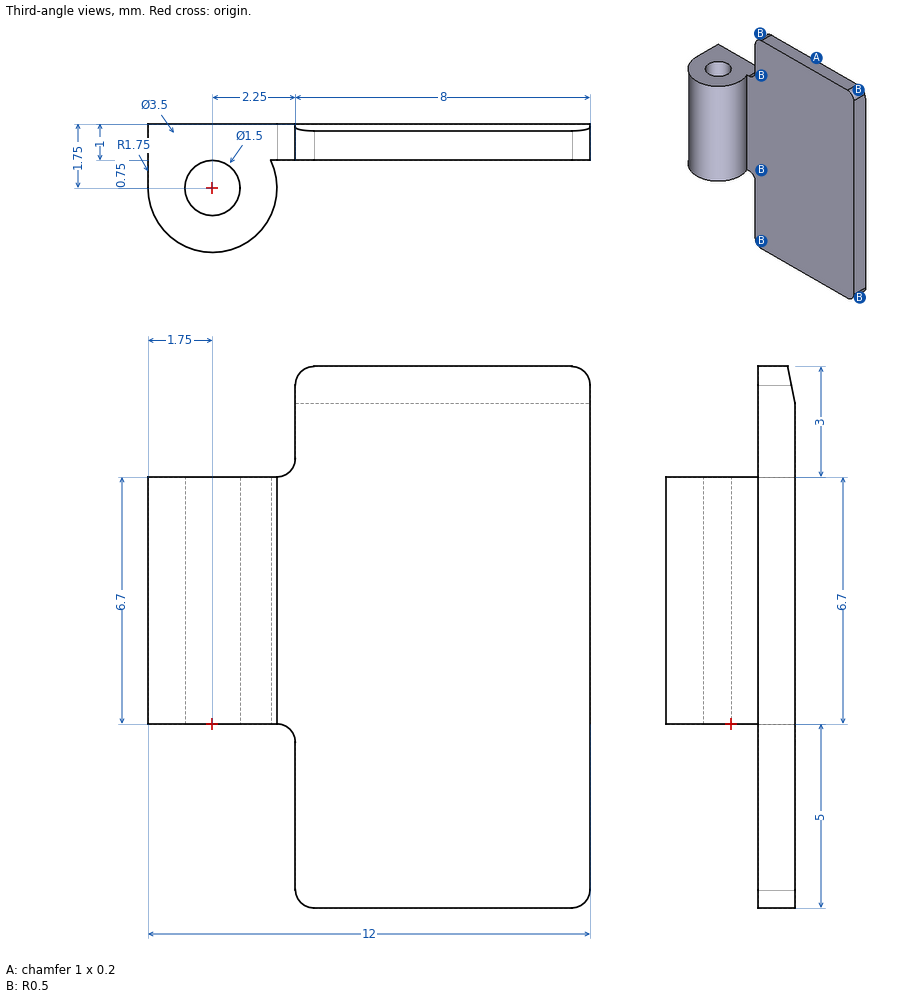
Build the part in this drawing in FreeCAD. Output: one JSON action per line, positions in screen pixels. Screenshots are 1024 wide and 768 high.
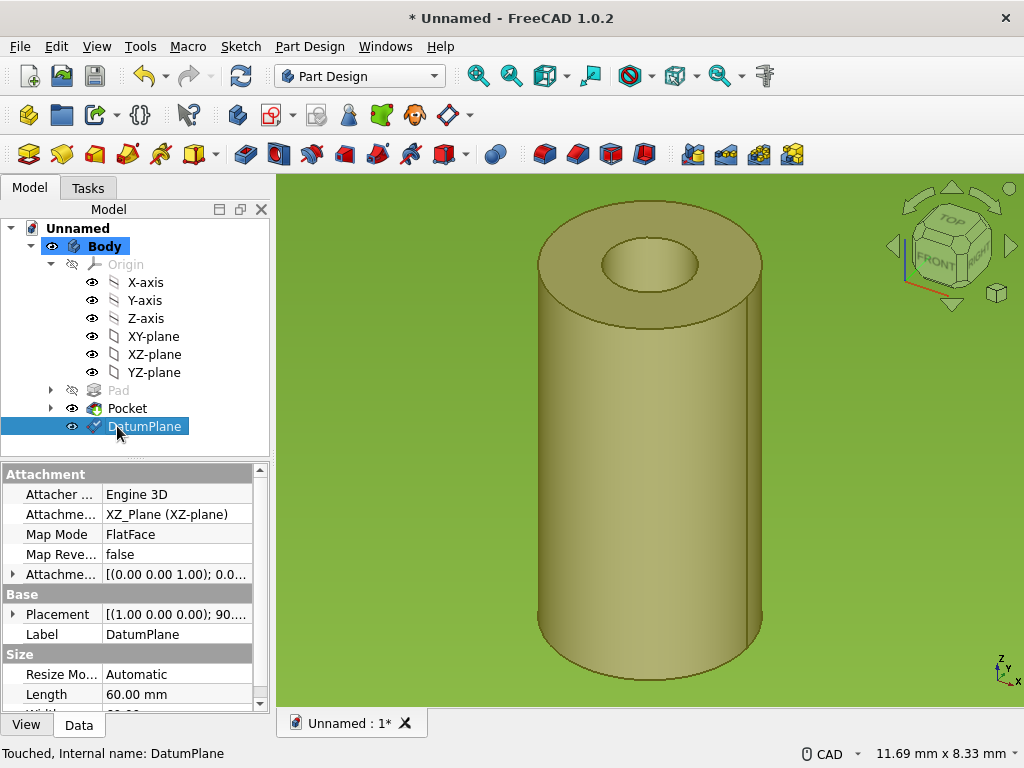
{"action": "left_click", "coordinate": [270, 116]}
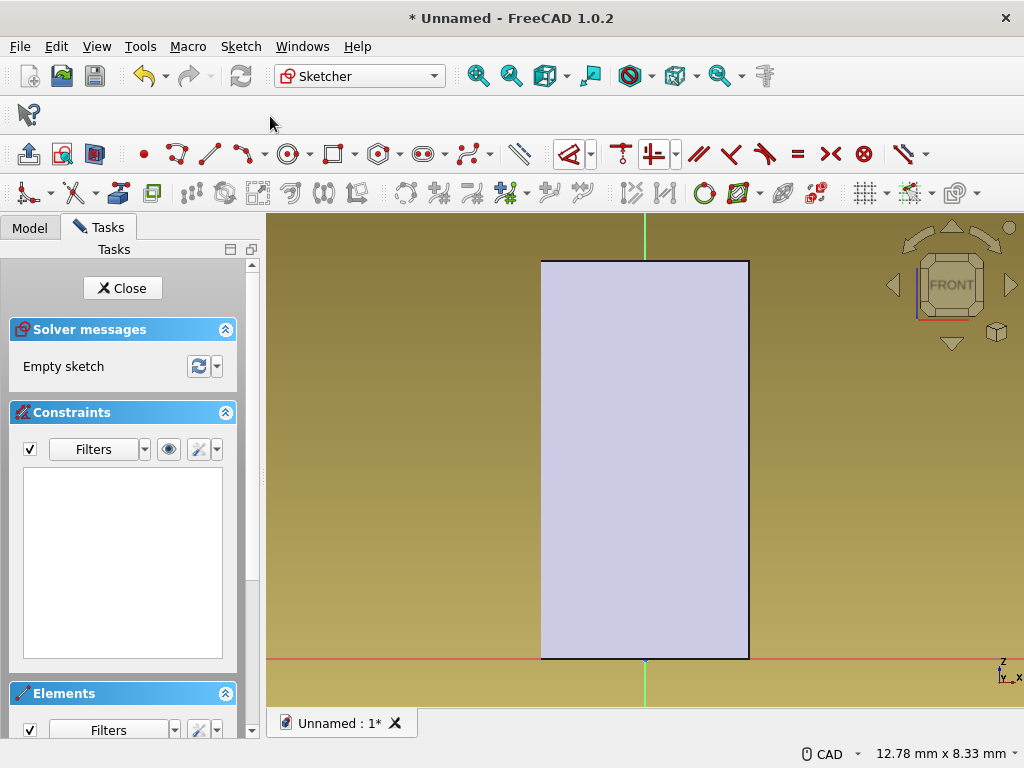
{"action": "key", "text": "q s"}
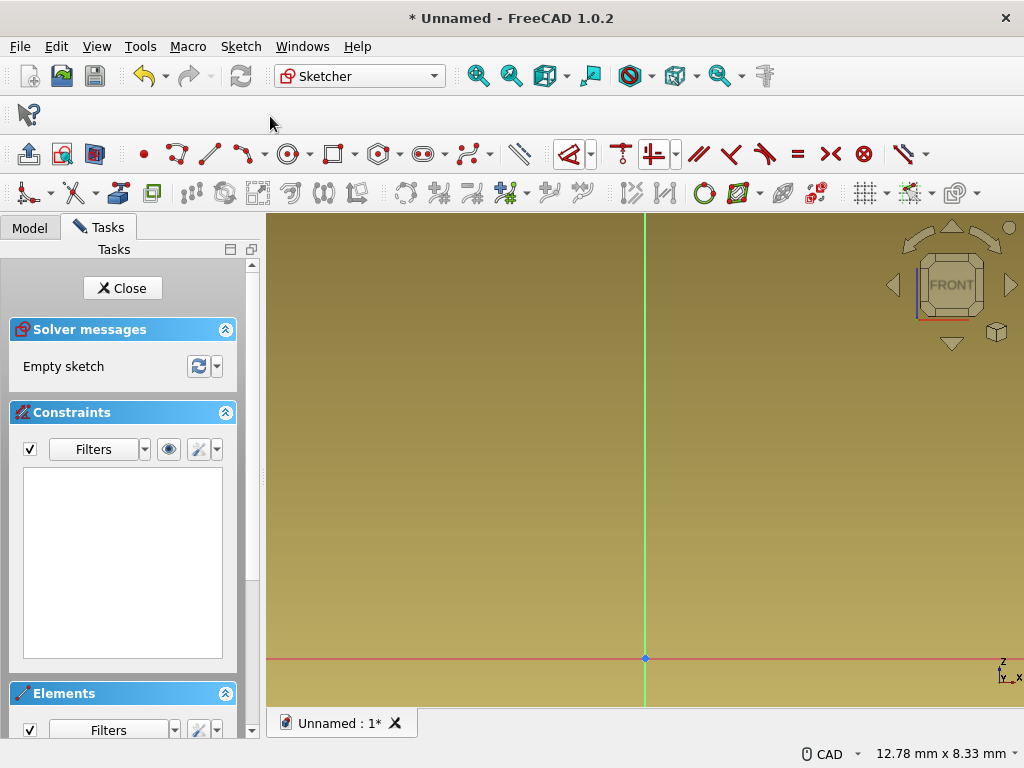
{"action": "scroll", "coordinate": [294, 460], "scroll_direction": "down", "scroll_amount": 3}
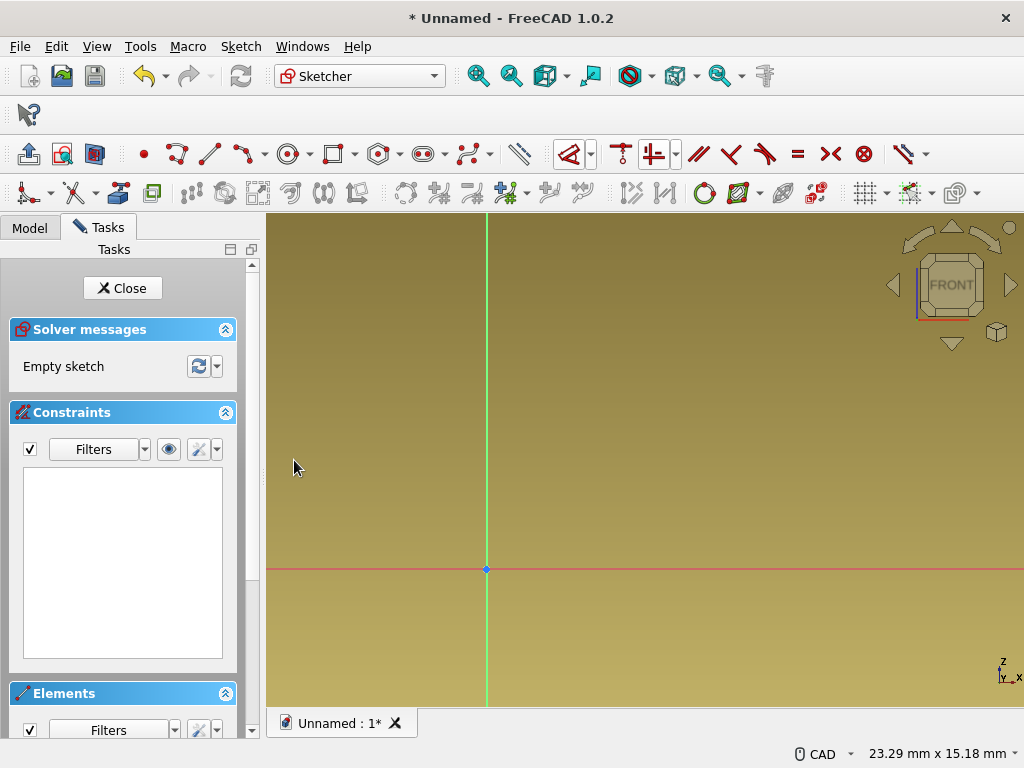
{"action": "left_click", "coordinate": [332, 154]}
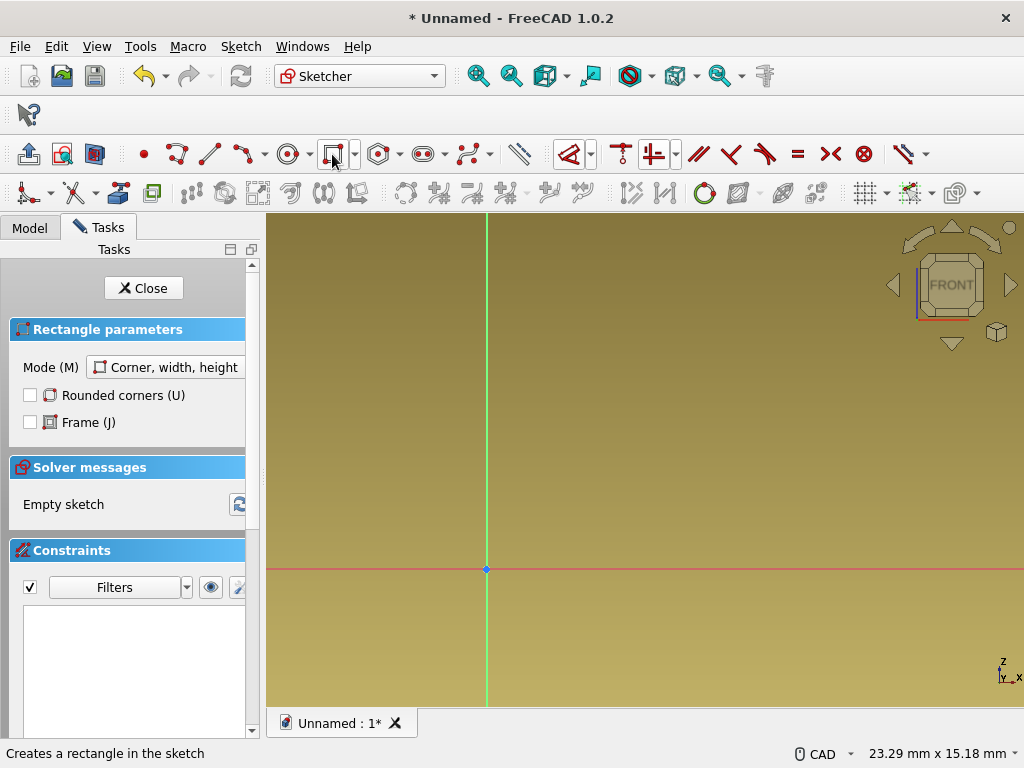
{"action": "left_click", "coordinate": [430, 351]}
{"action": "left_click", "coordinate": [820, 569]}
{"action": "key", "text": "Escape"}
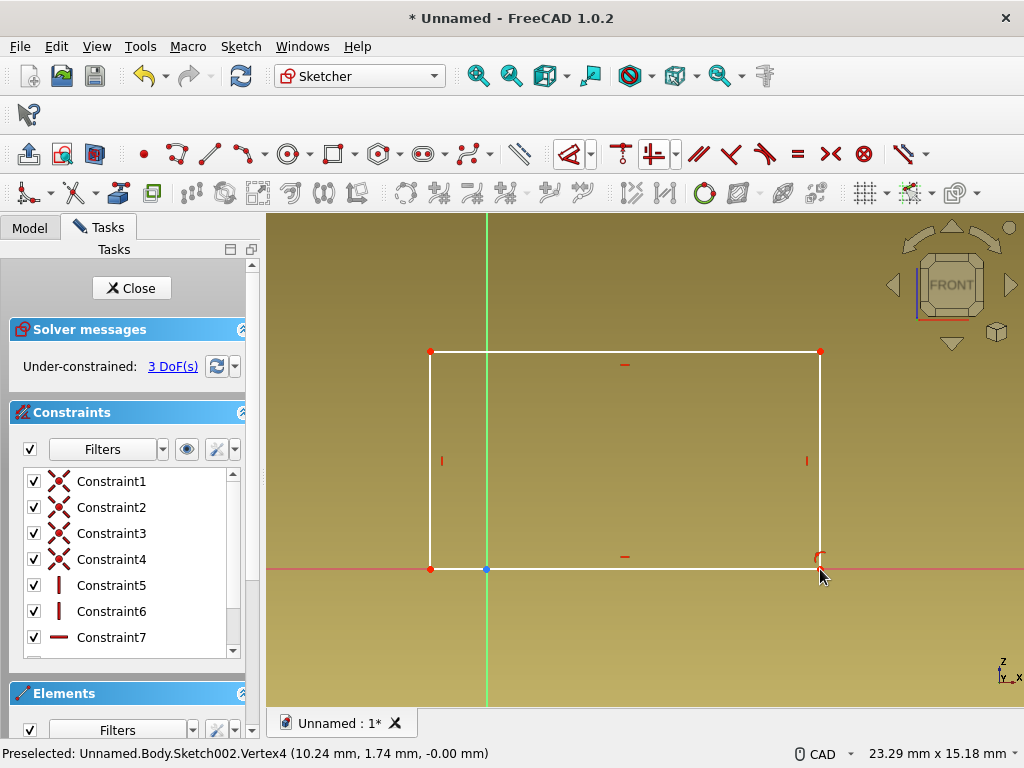
{"action": "left_click", "coordinate": [547, 569]}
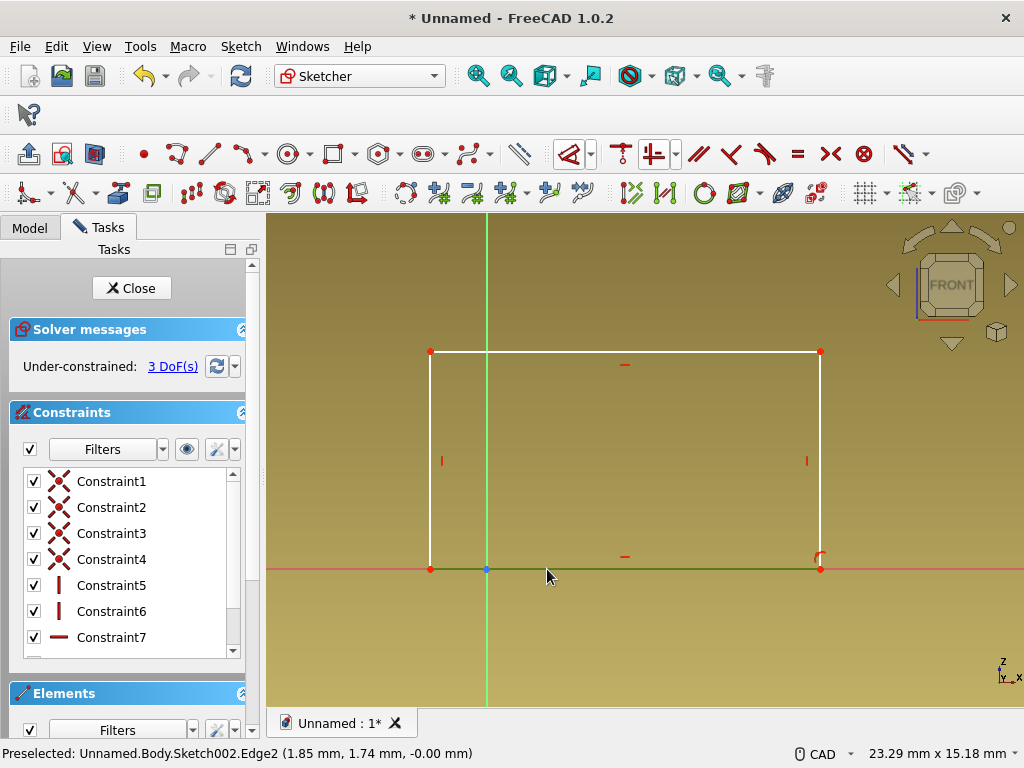
{"action": "left_click", "coordinate": [590, 154]}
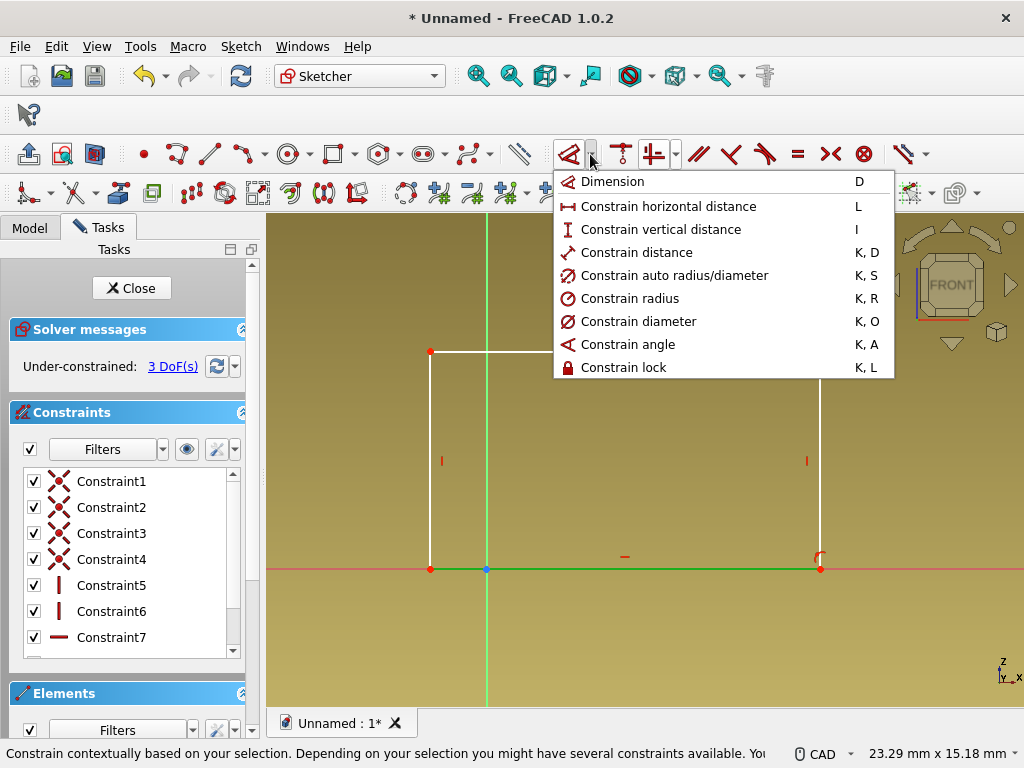
{"action": "left_click", "coordinate": [724, 206]}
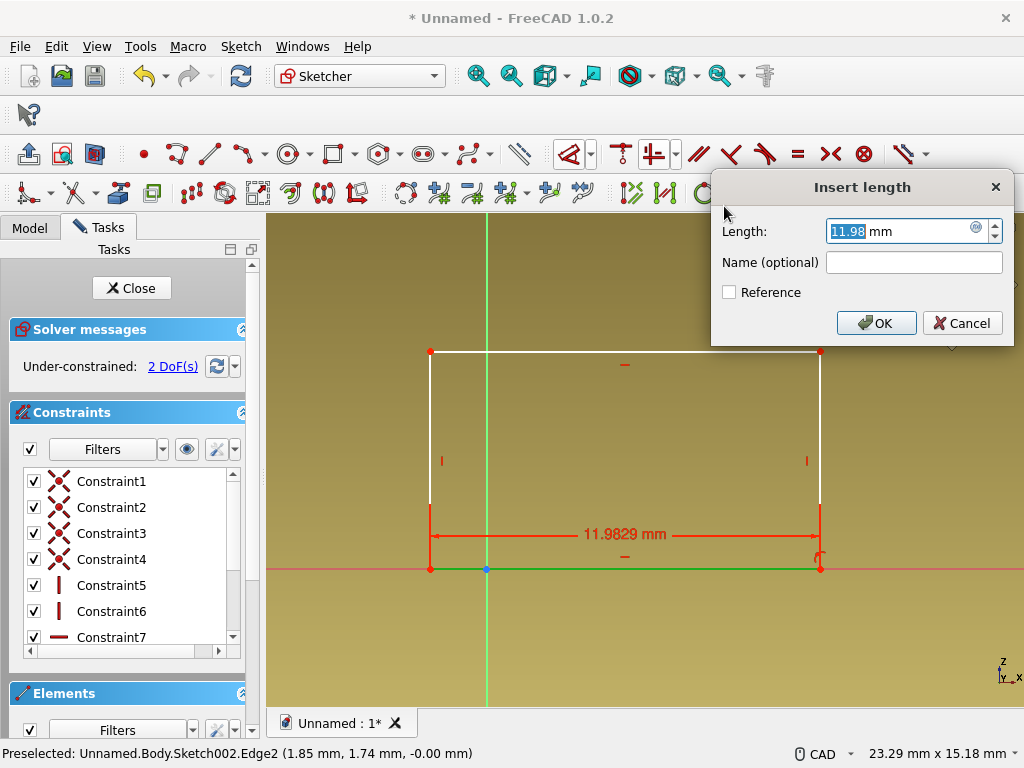
{"action": "type", "text": "12"}
{"action": "key", "text": "Return"}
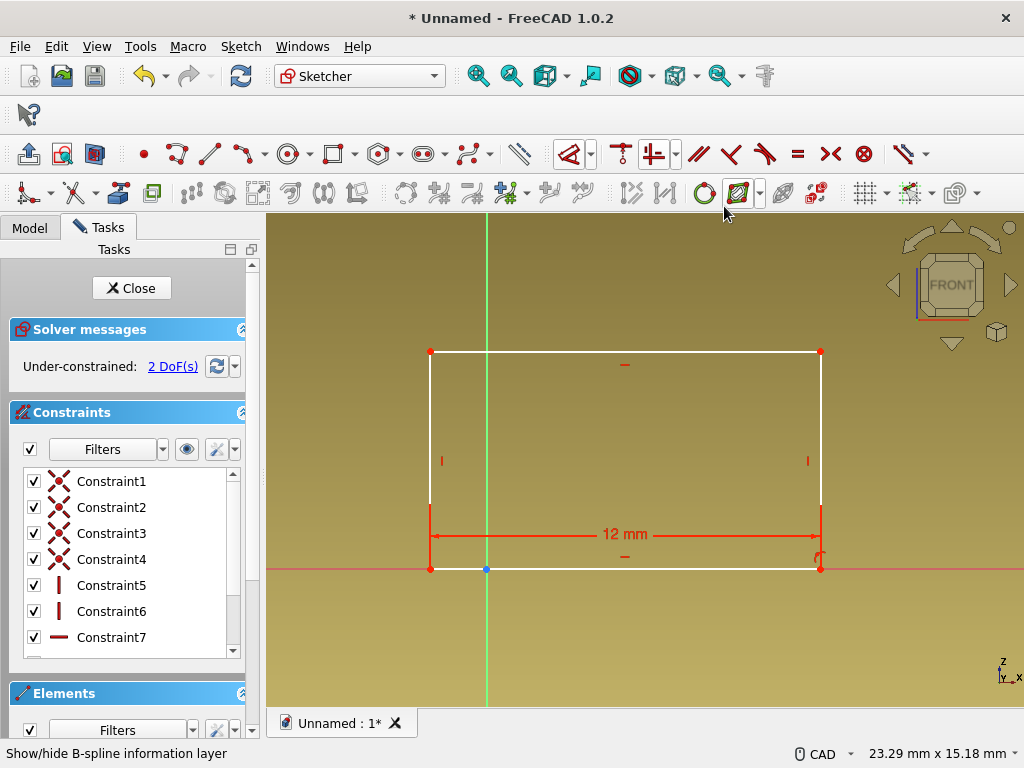
{"action": "left_click", "coordinate": [430, 417]}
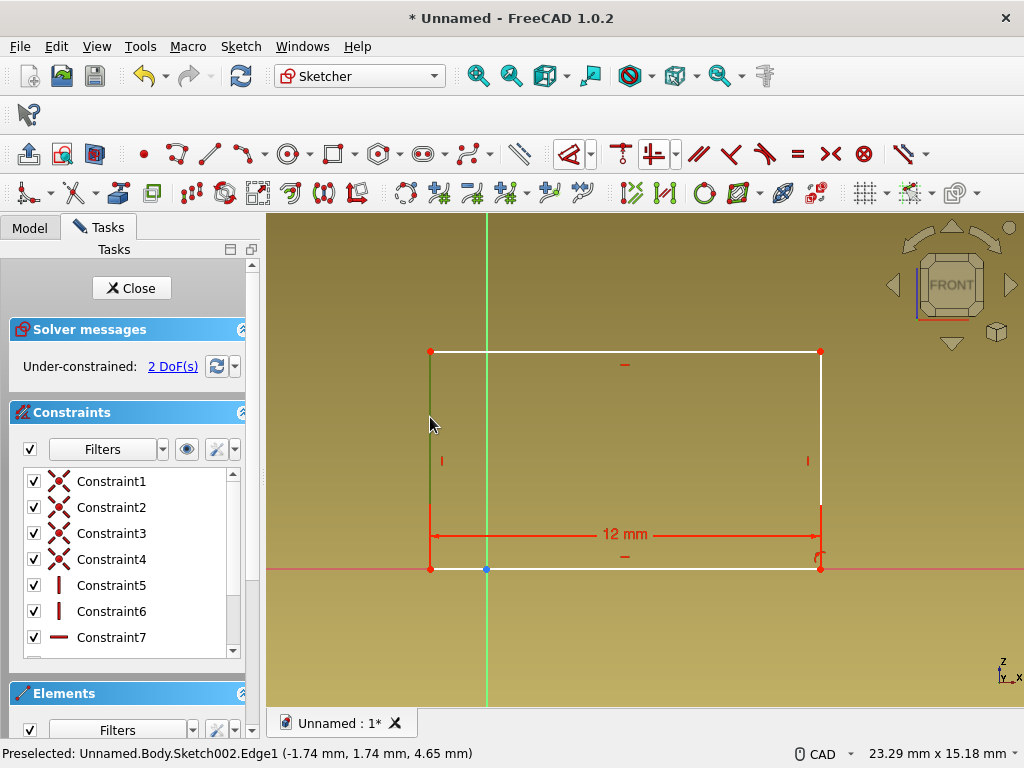
{"action": "left_click", "coordinate": [590, 154]}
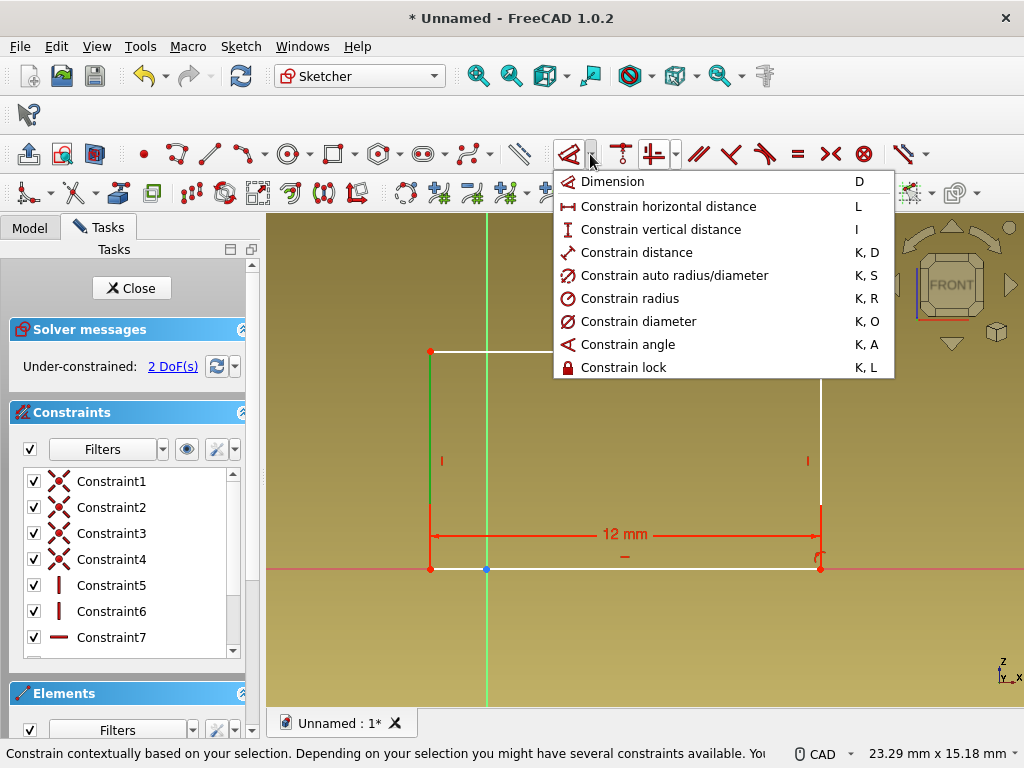
{"action": "left_click", "coordinate": [724, 230]}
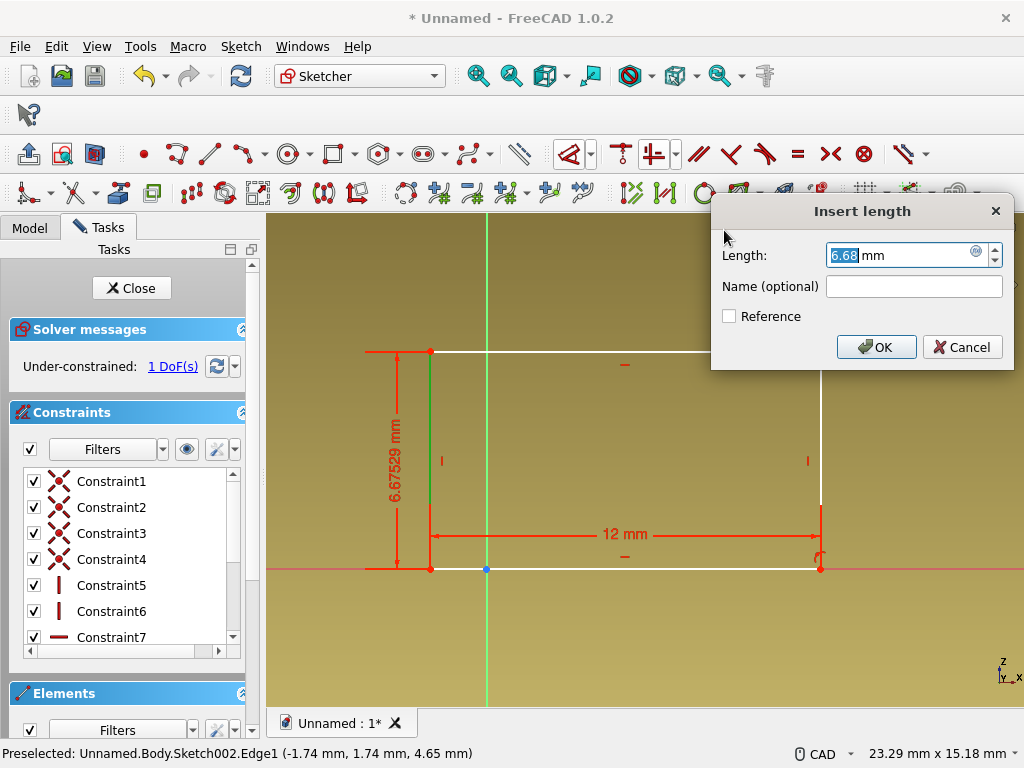
{"action": "type", "text": "6.7"}
{"action": "key", "text": "Return"}